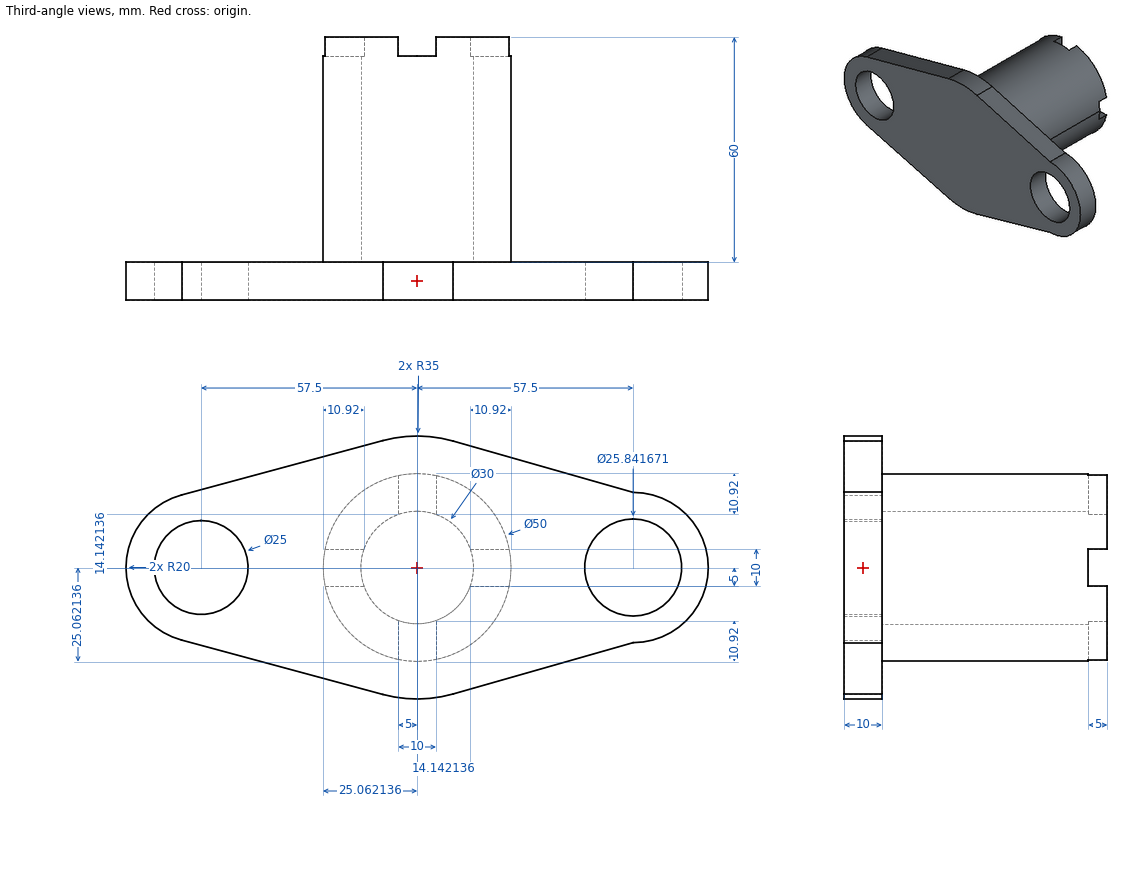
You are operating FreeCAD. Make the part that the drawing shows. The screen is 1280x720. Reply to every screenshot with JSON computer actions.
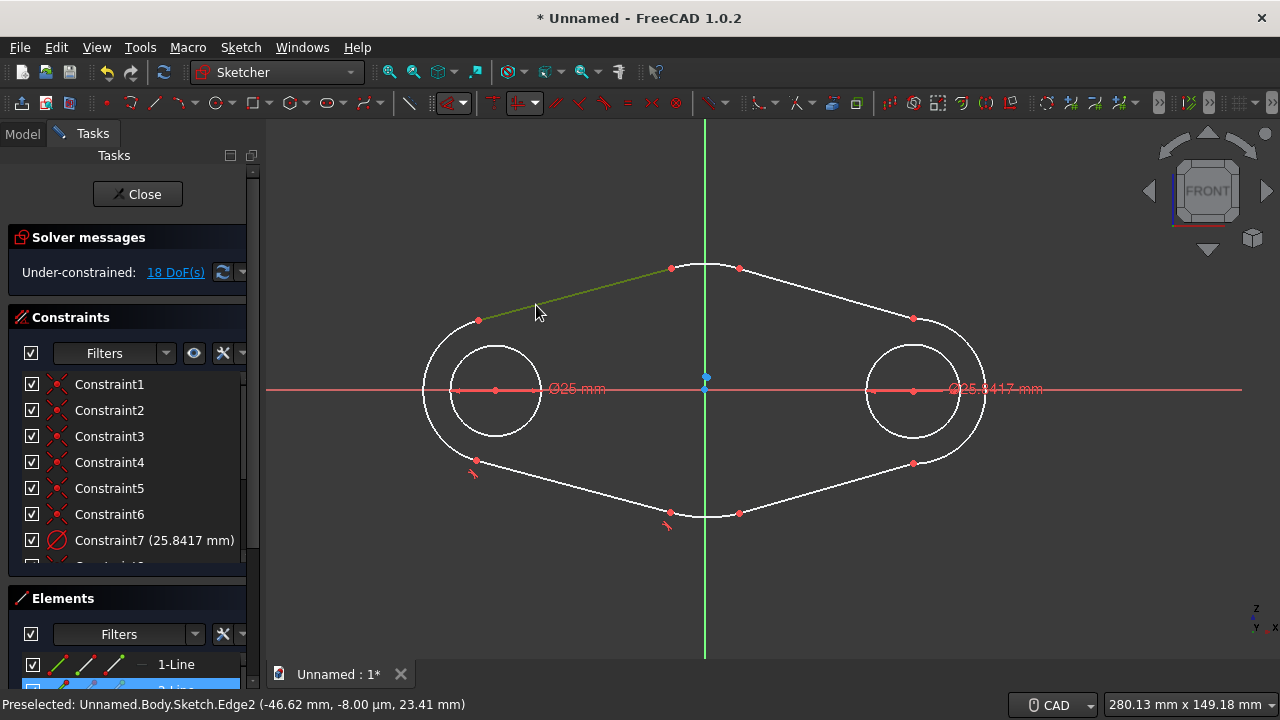
{"action": "left_click", "coordinate": [433, 354]}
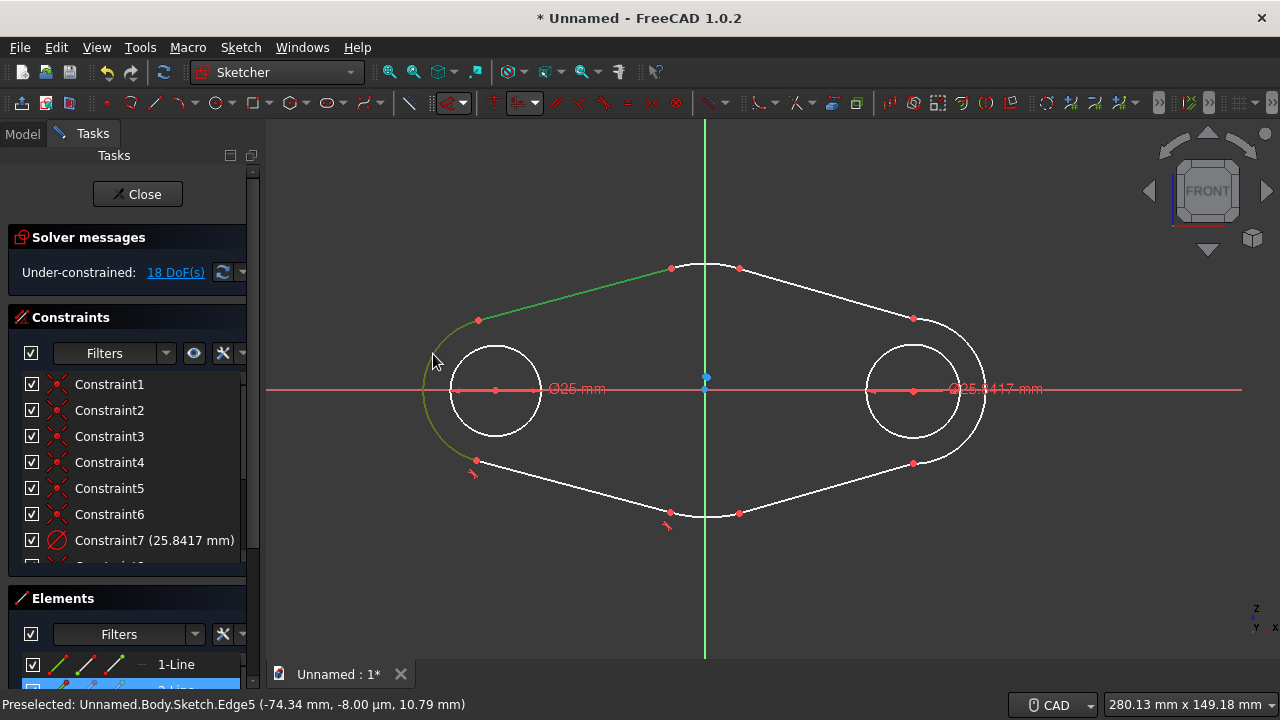
{"action": "key", "text": "t"}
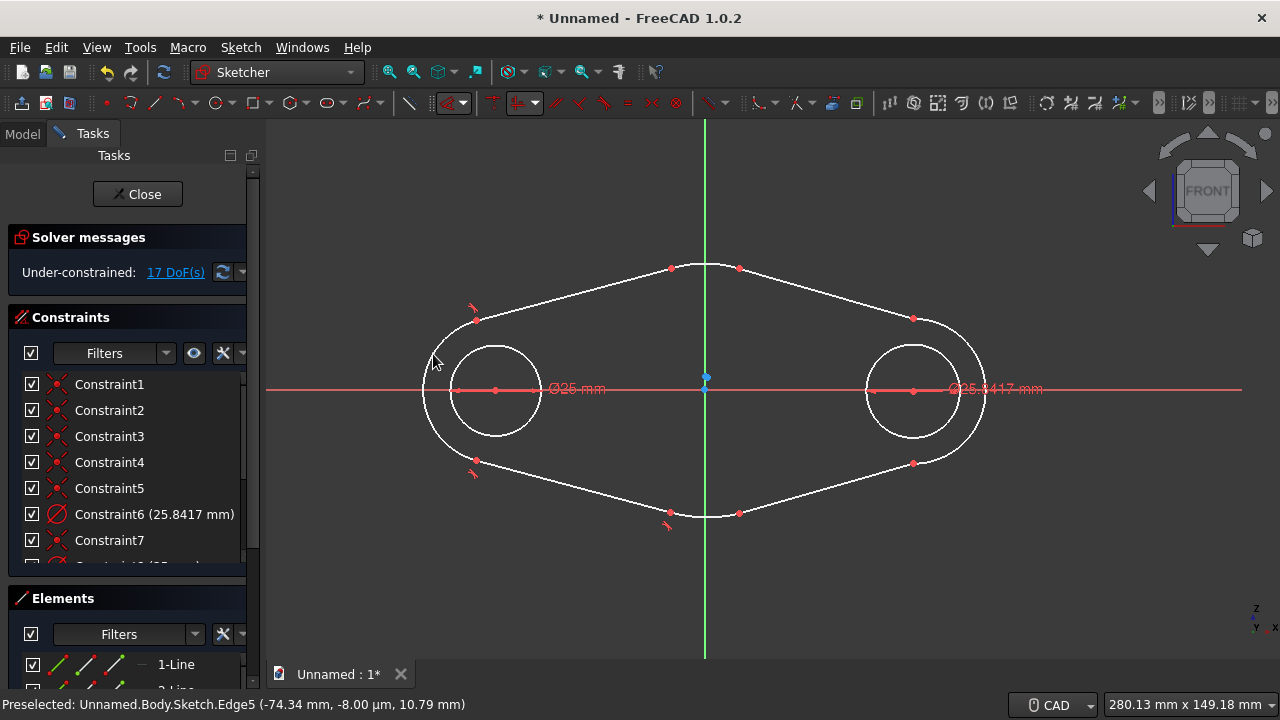
{"action": "left_click", "coordinate": [535, 305]}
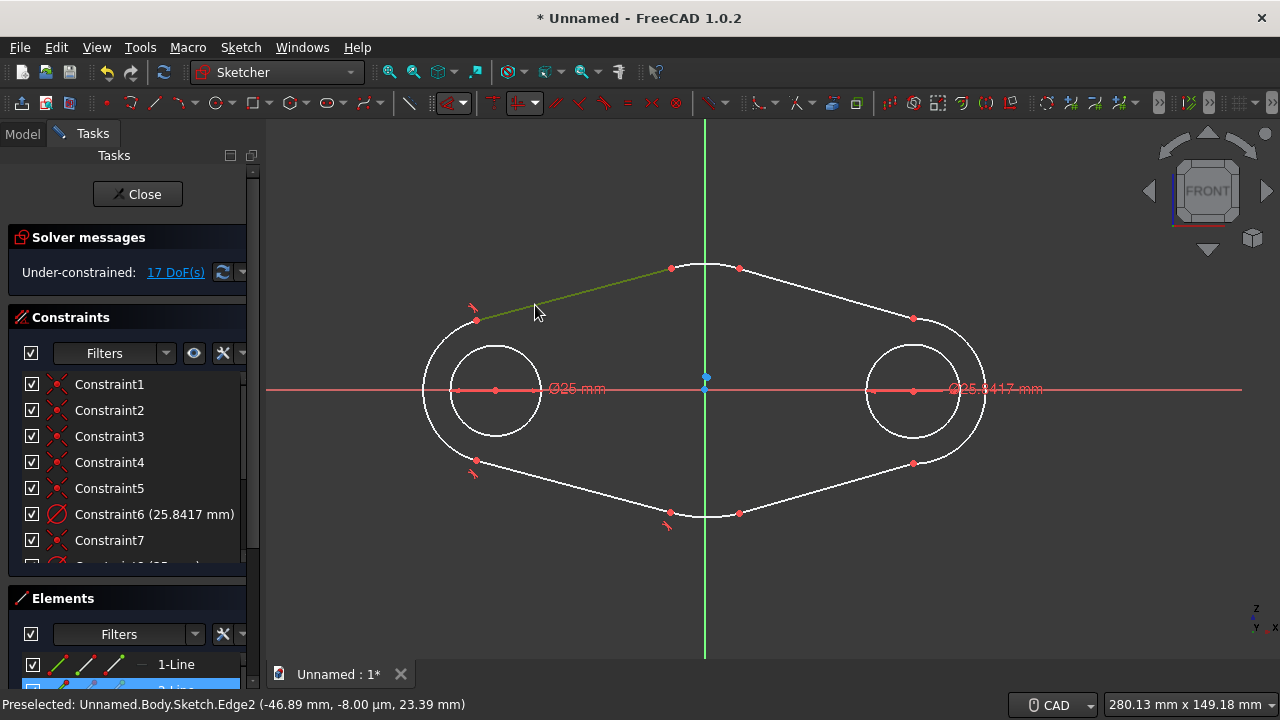
{"action": "left_click", "coordinate": [719, 264]}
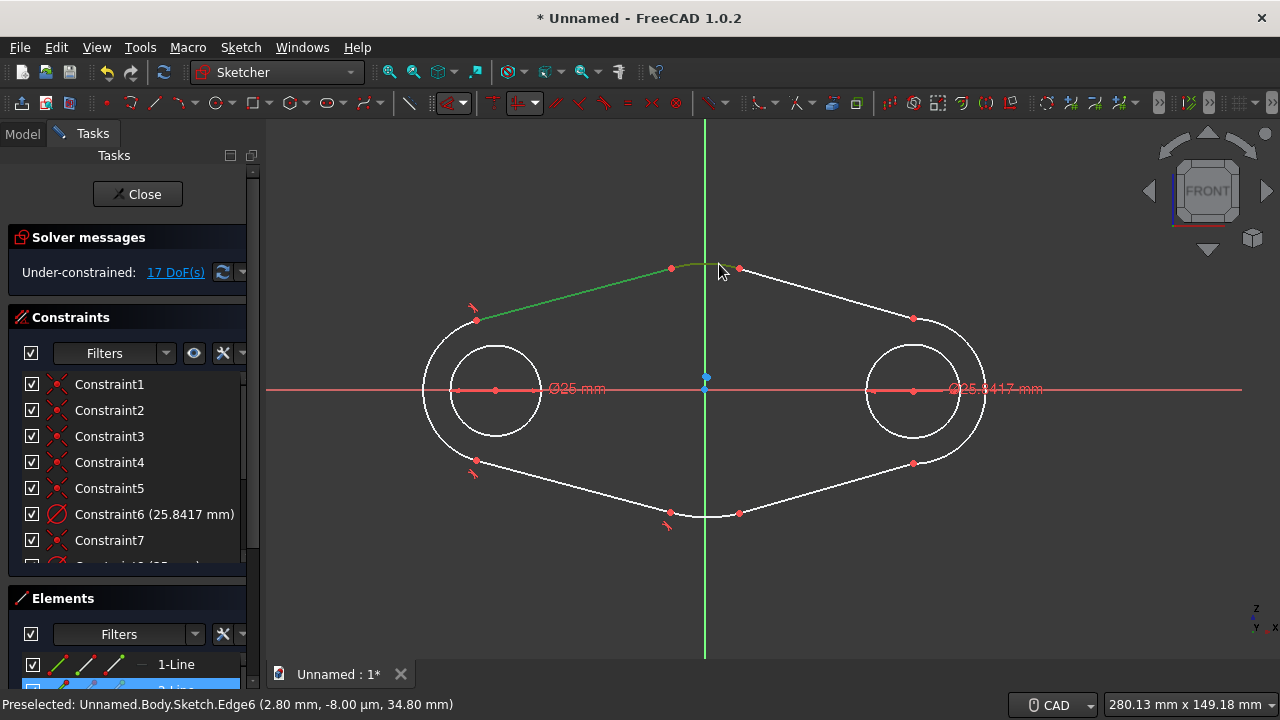
{"action": "key", "text": "t"}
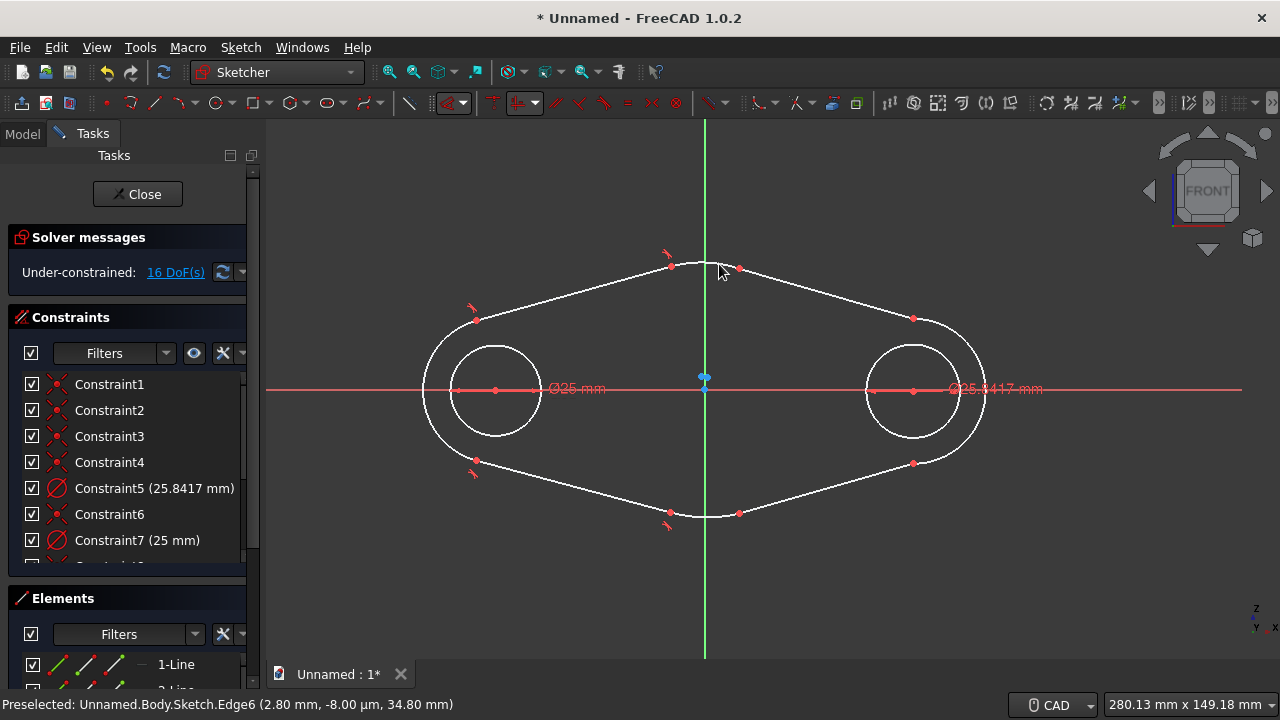
{"action": "left_click", "coordinate": [791, 284]}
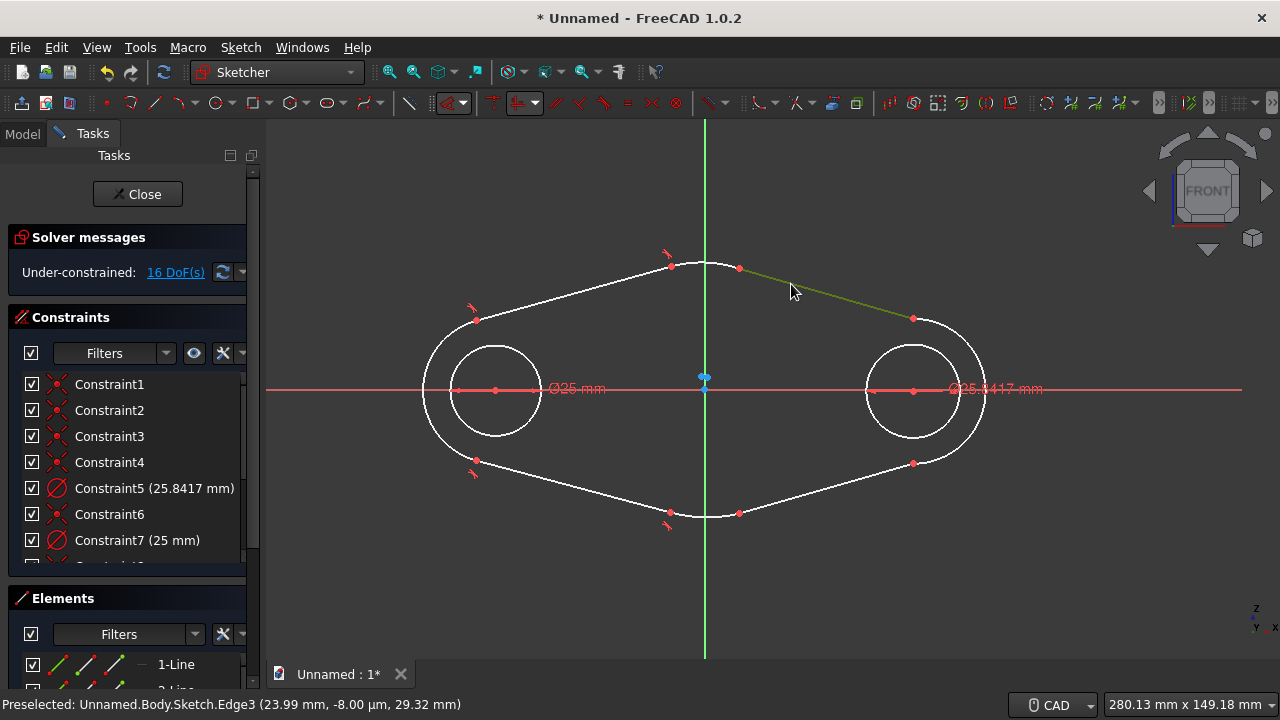
{"action": "left_click", "coordinate": [719, 264]}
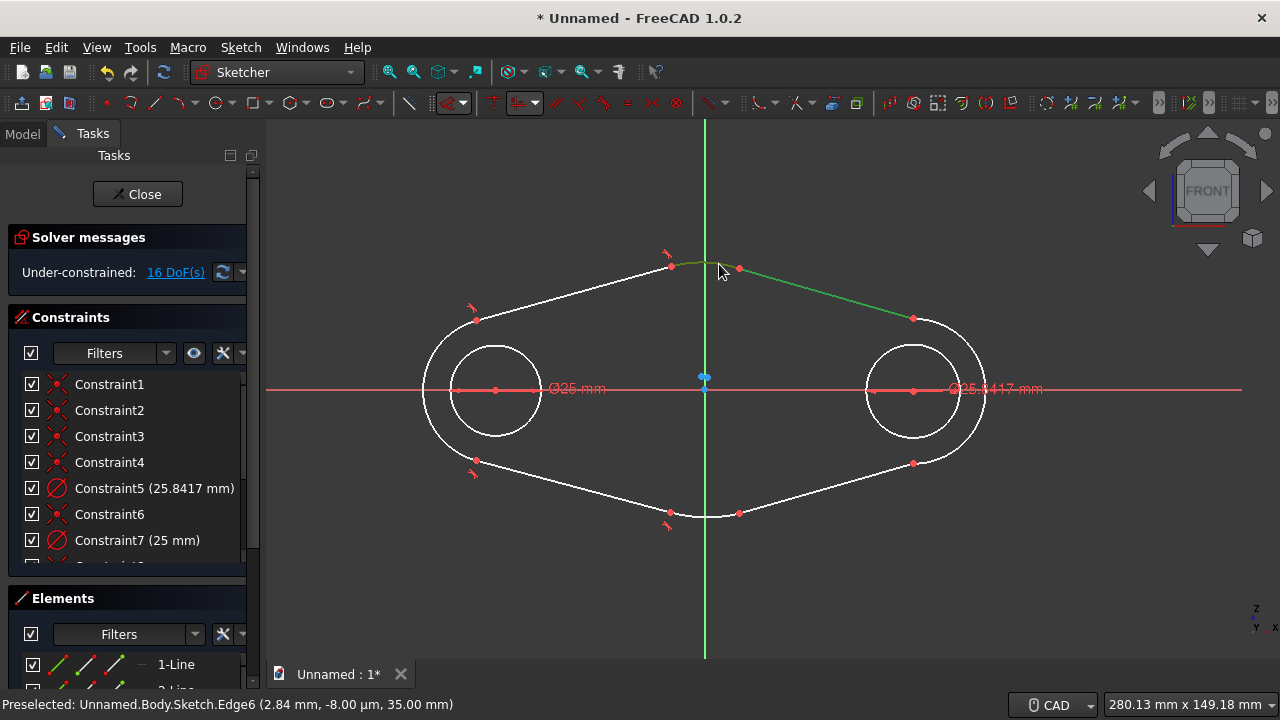
{"action": "left_click", "coordinate": [604, 104]}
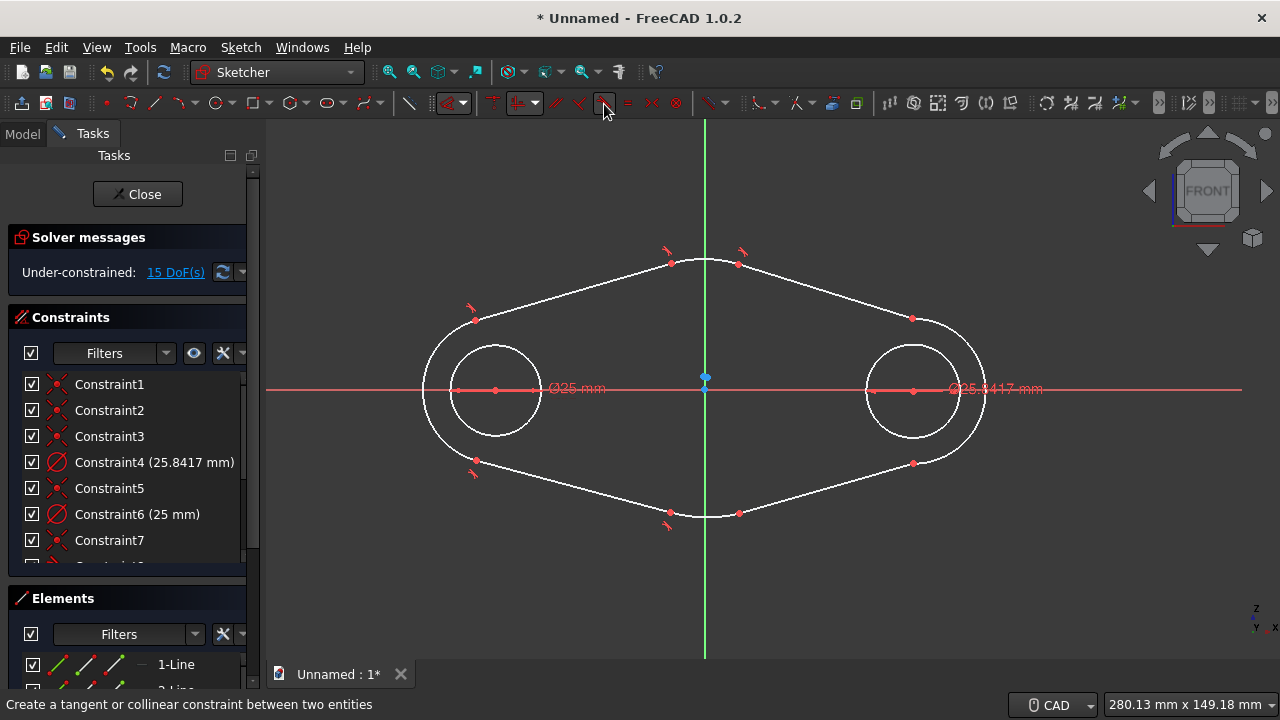
{"action": "left_click", "coordinate": [861, 479]}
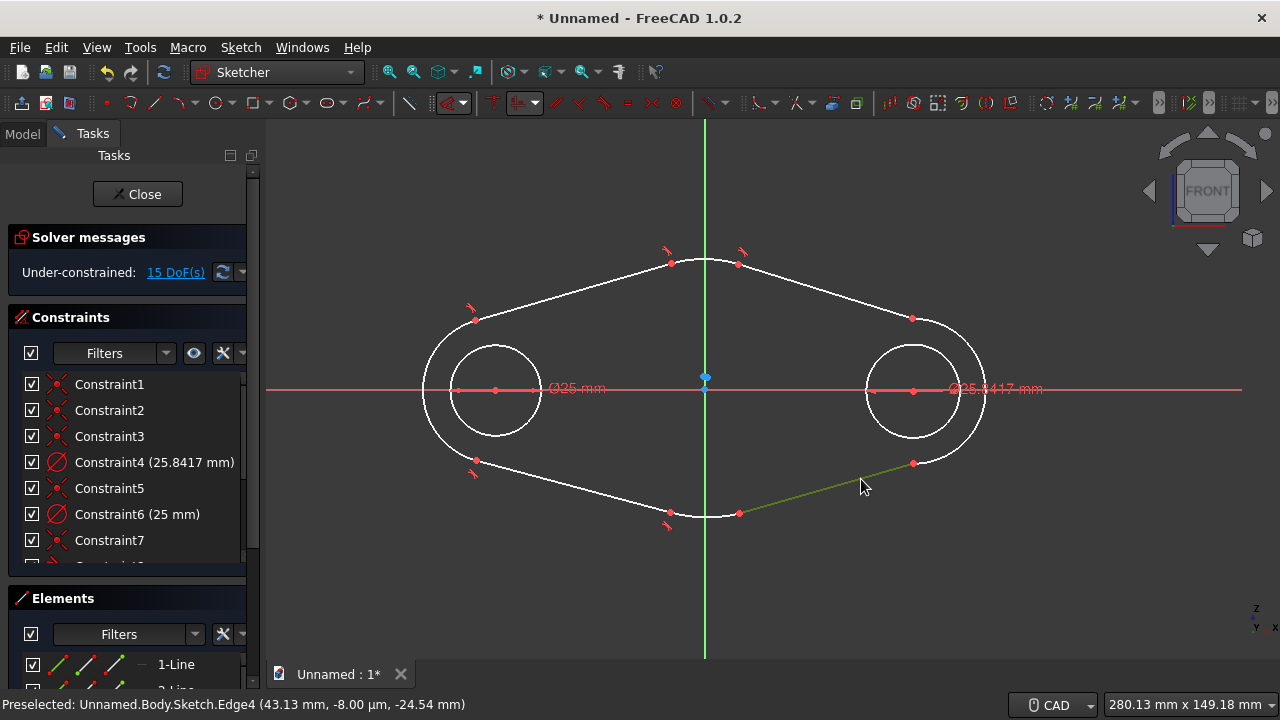
{"action": "left_click", "coordinate": [691, 516]}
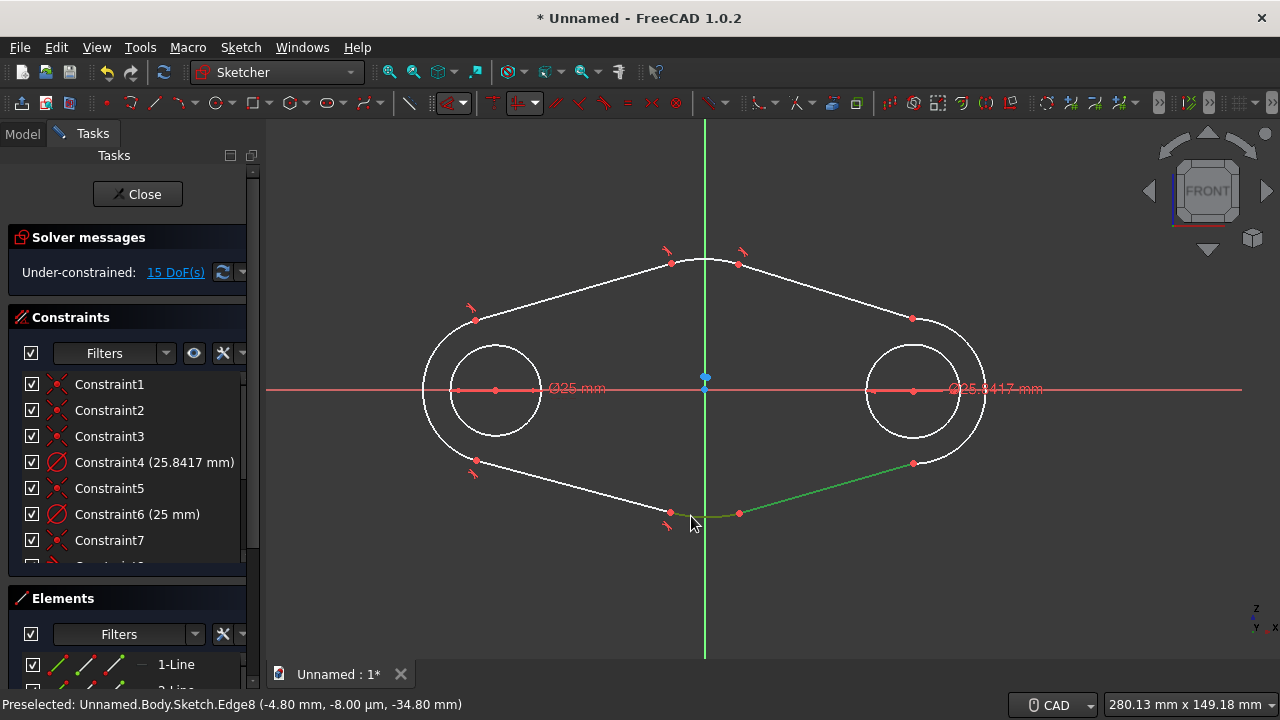
{"action": "key", "text": "t"}